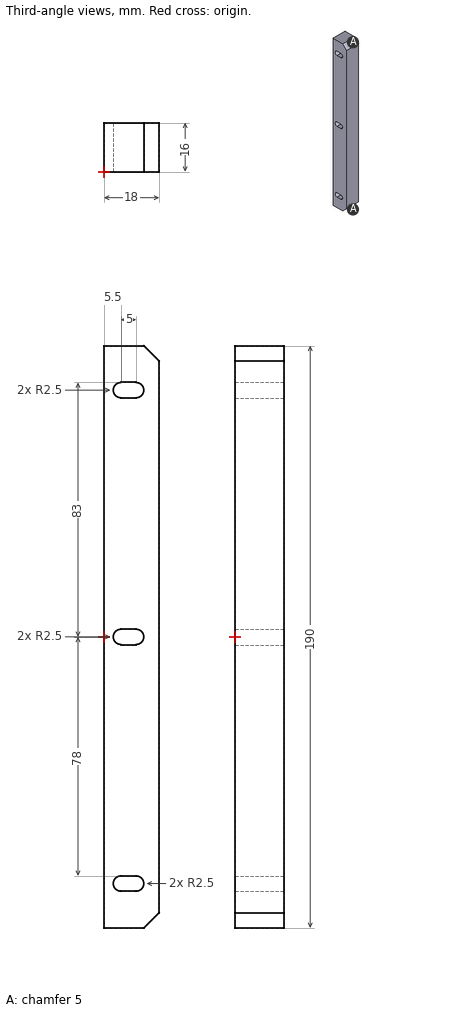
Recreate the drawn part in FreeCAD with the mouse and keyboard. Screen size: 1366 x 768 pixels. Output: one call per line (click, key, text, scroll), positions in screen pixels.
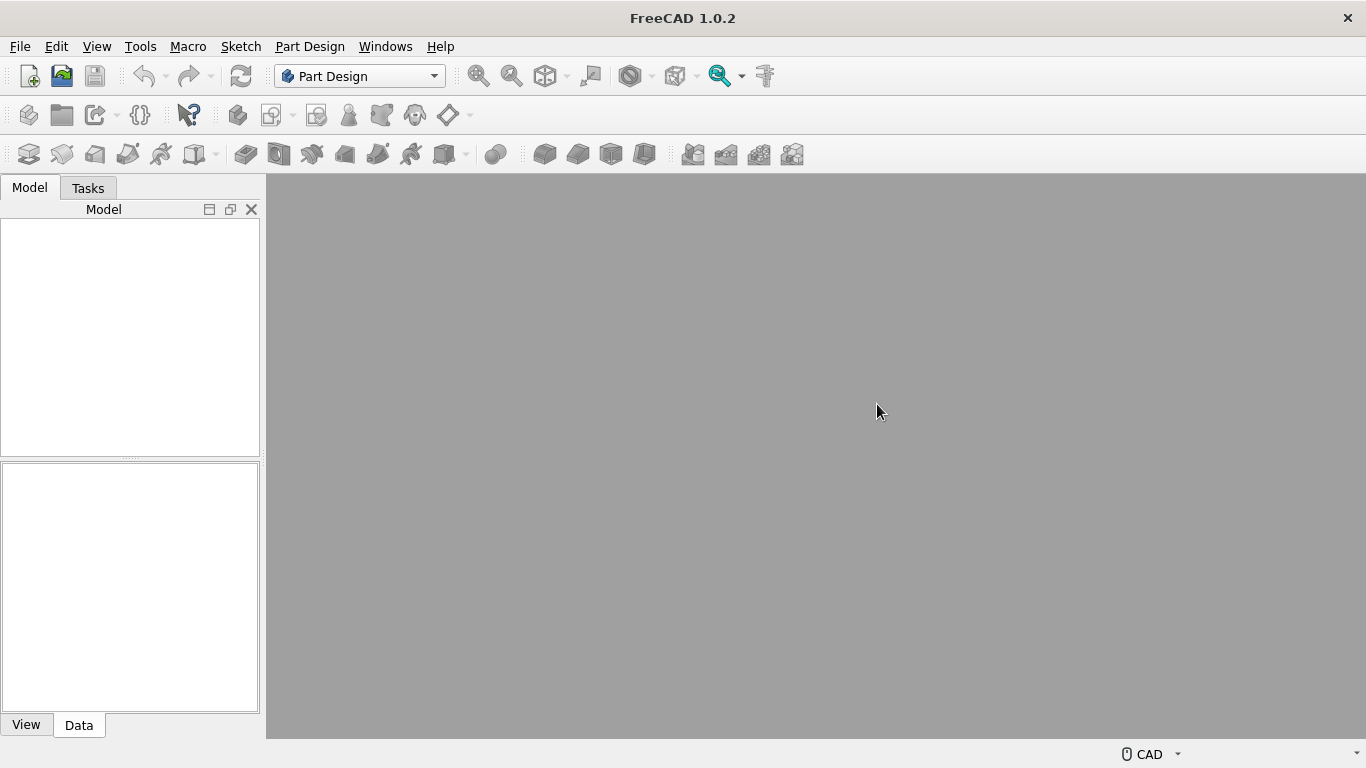
click(29, 76)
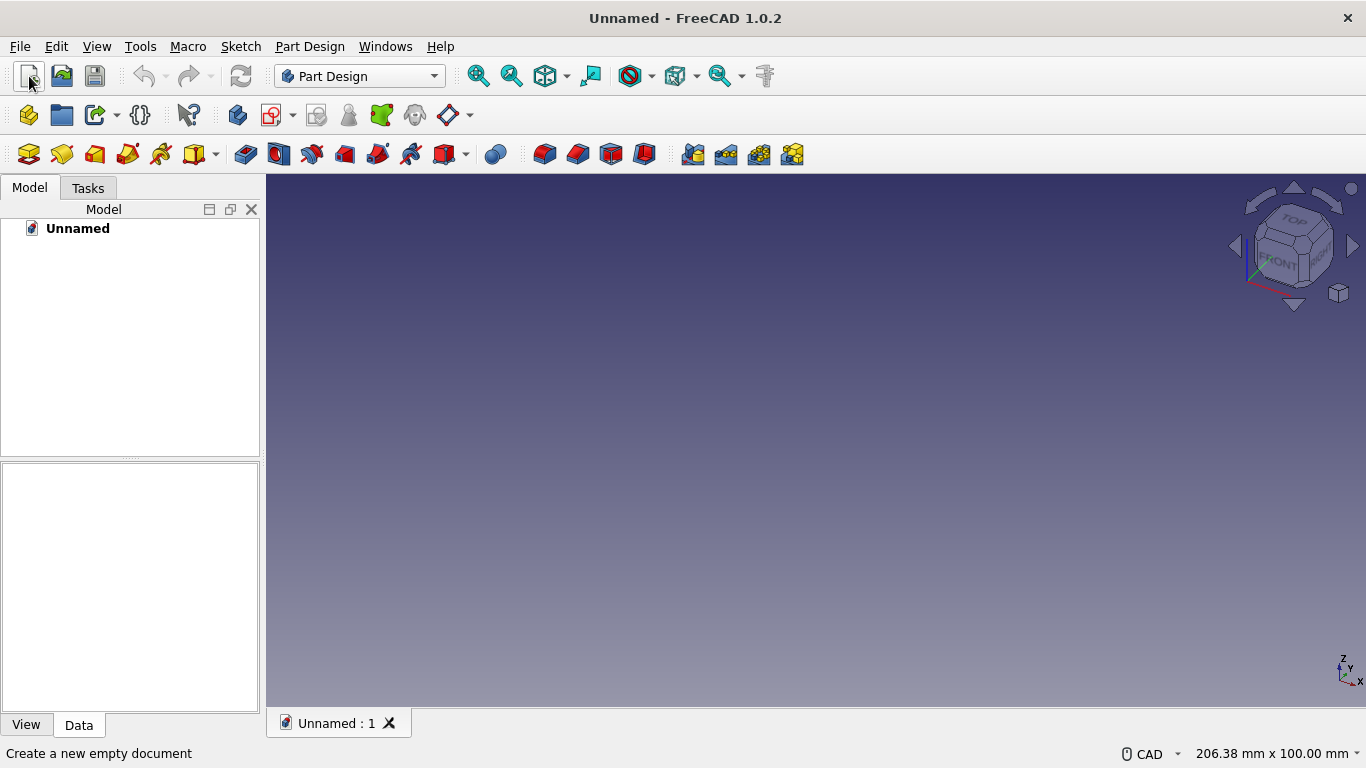
click(270, 116)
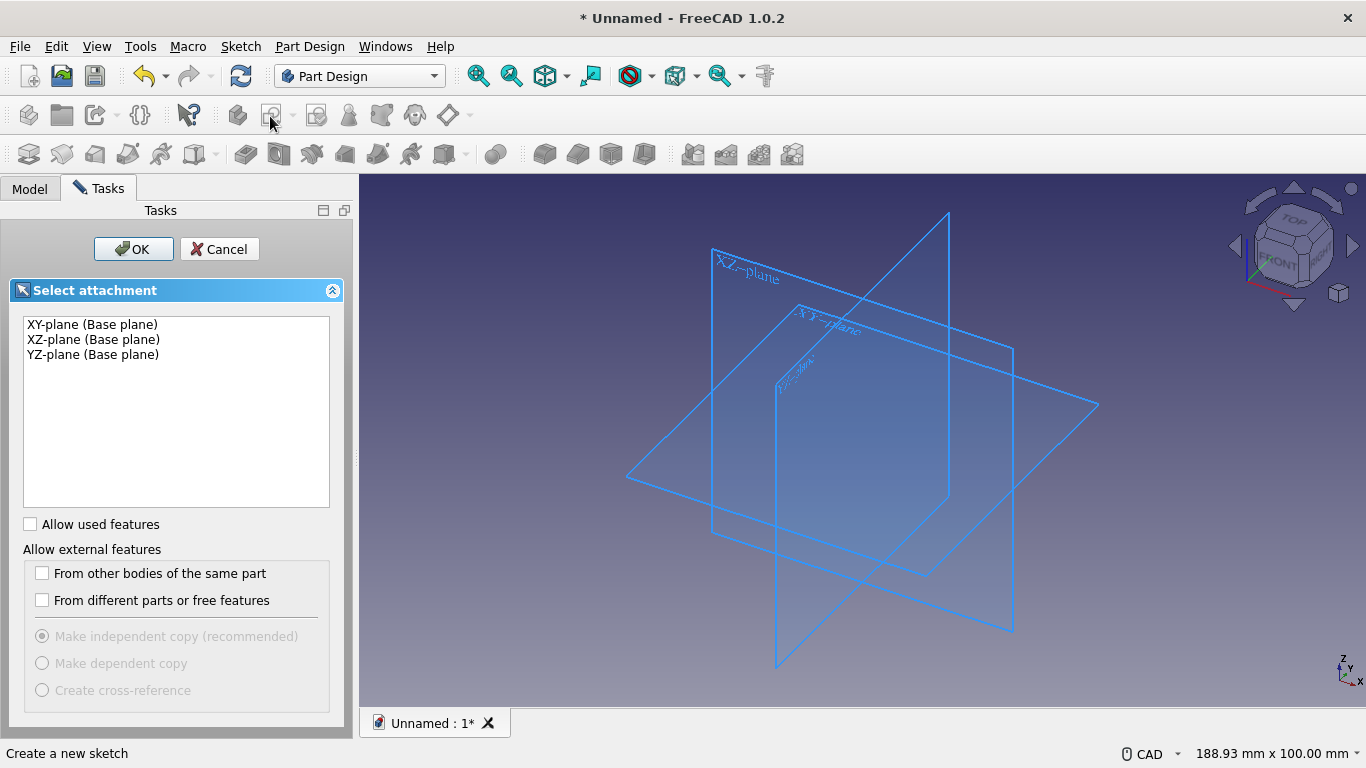
click(84, 324)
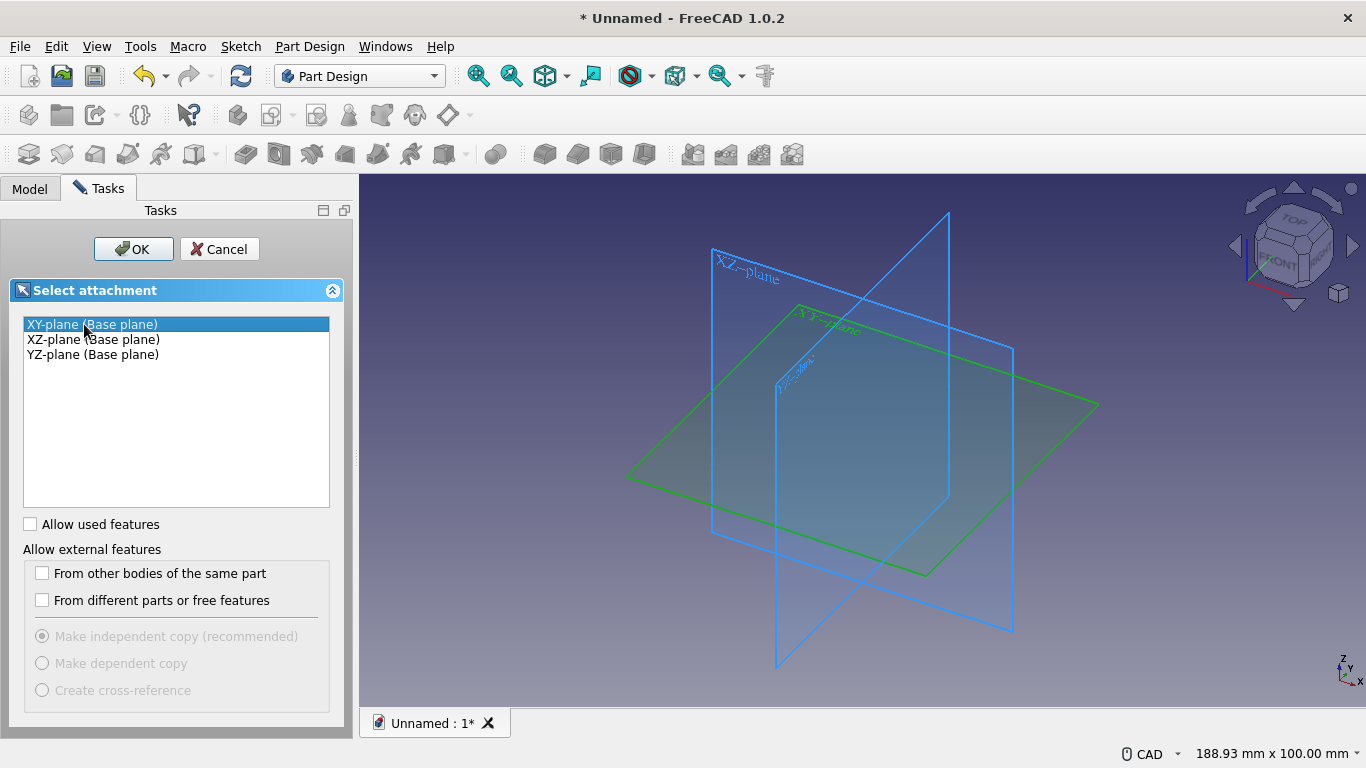
click(134, 249)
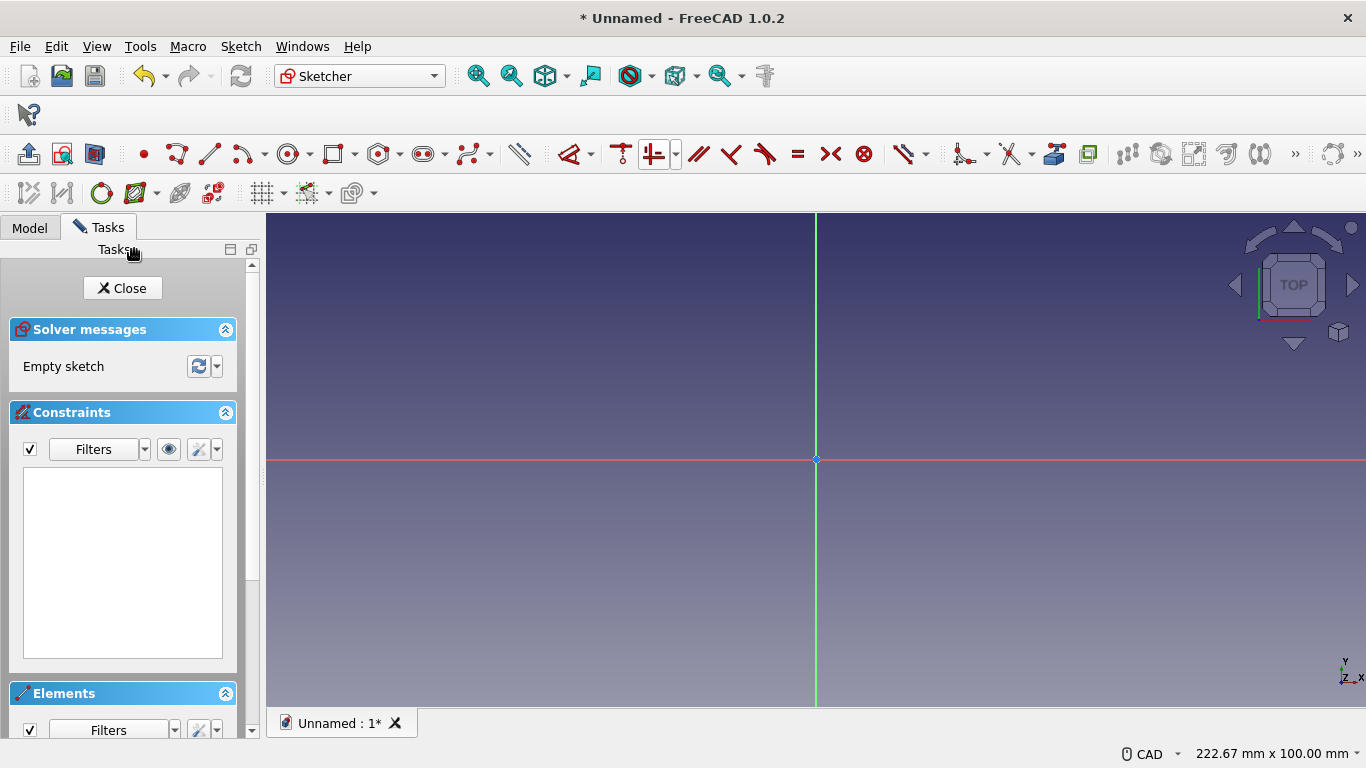
scroll(897, 408, up, 7)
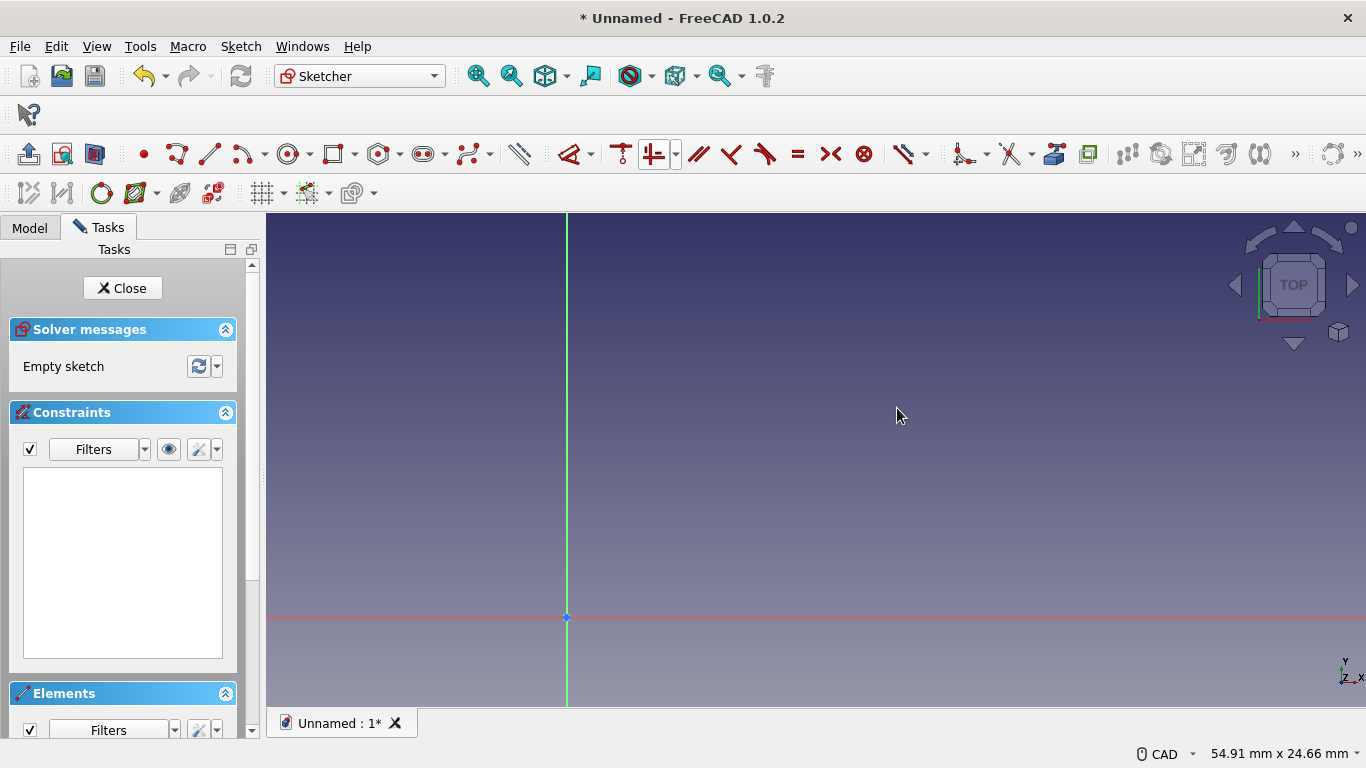
key(g)
key(r)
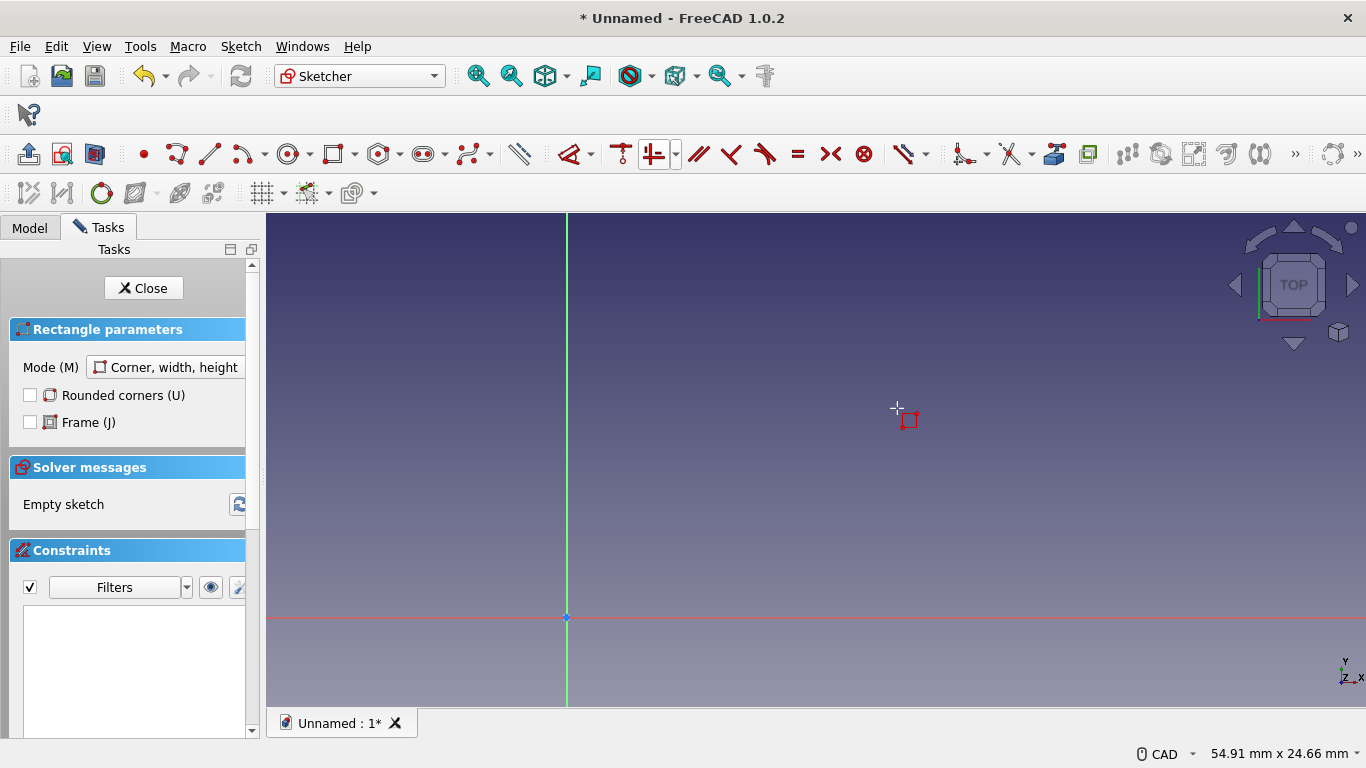
click(567, 618)
click(927, 297)
key(Escape)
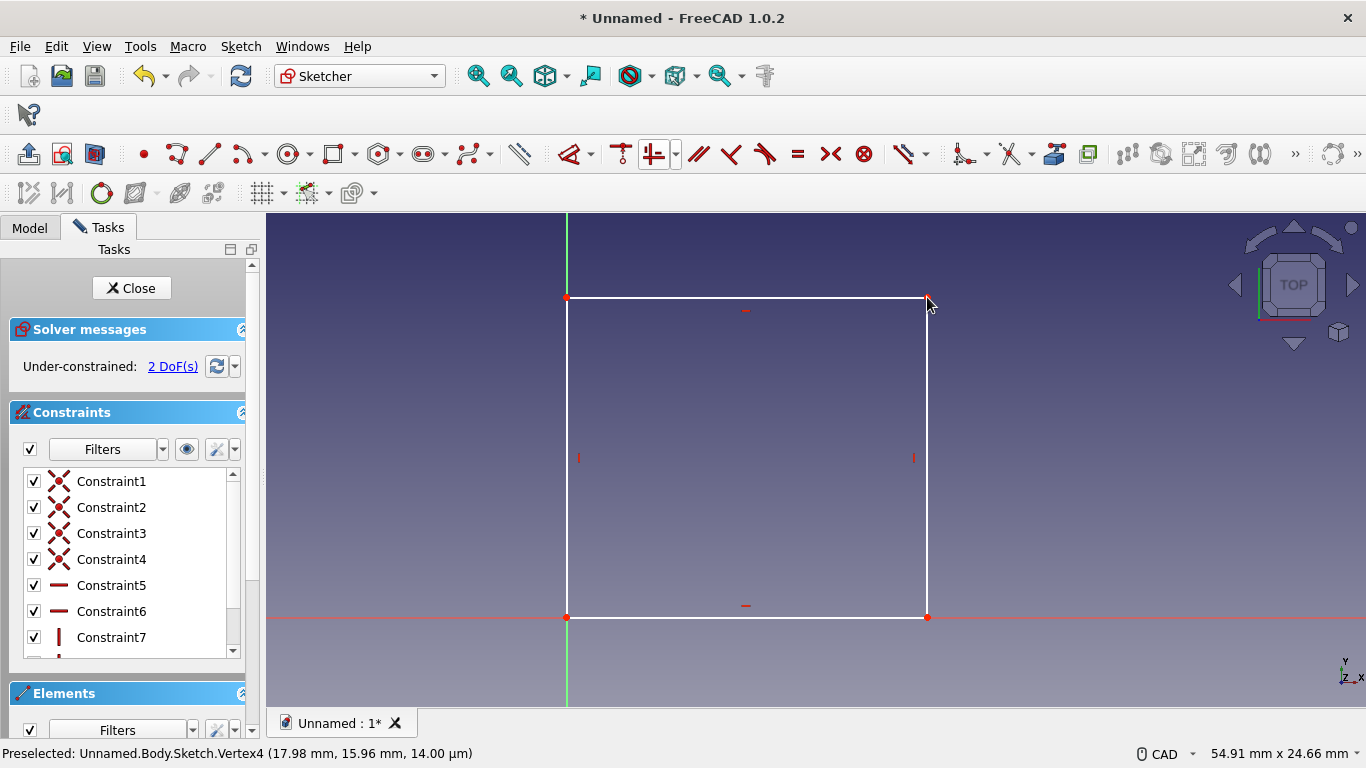
click(568, 154)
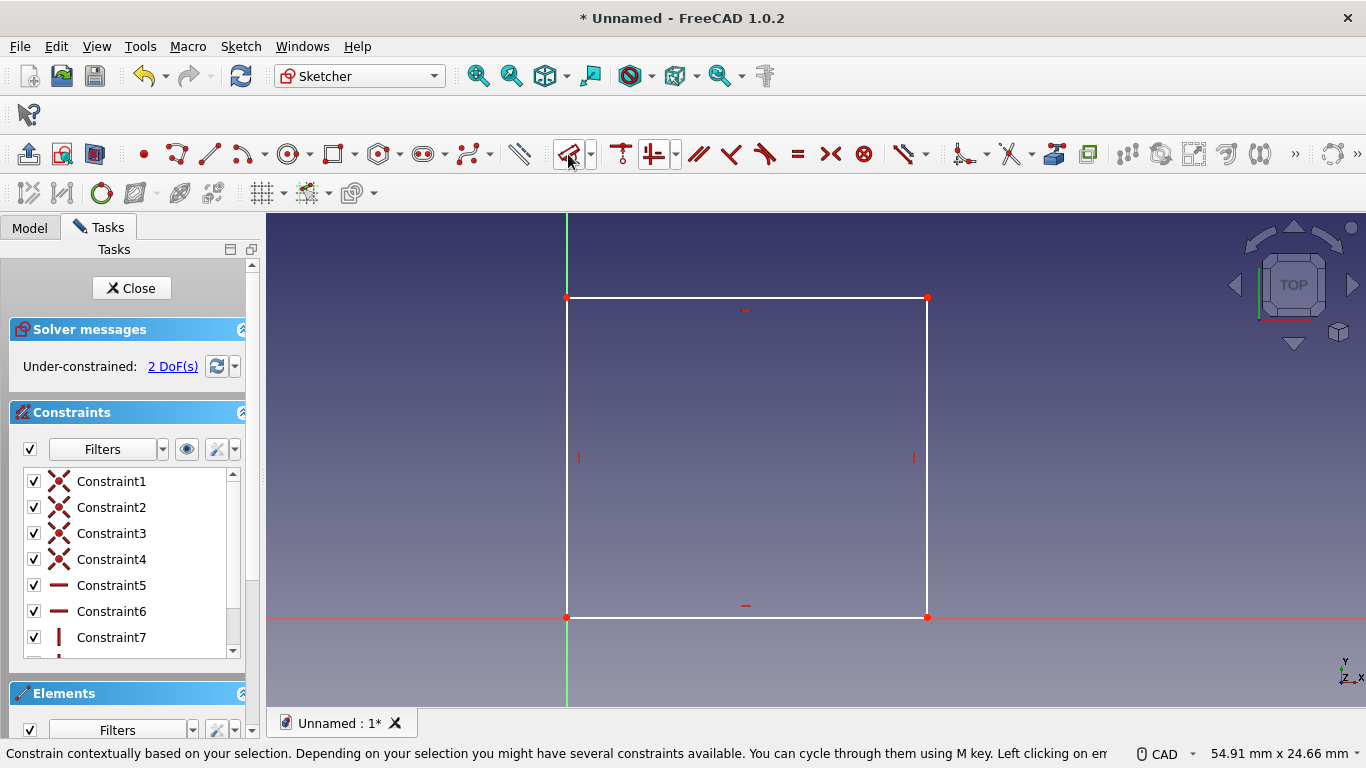
click(675, 618)
click(747, 652)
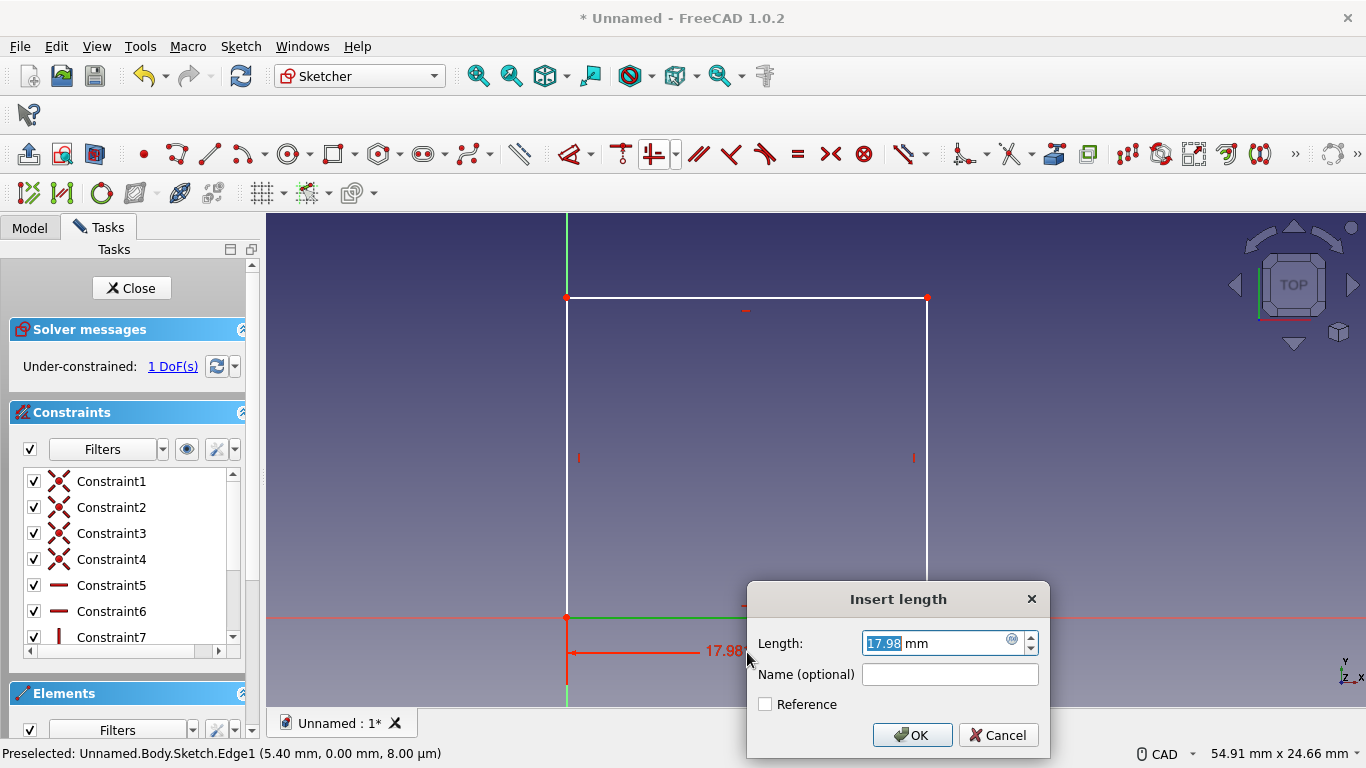
text(18)
key(Return)